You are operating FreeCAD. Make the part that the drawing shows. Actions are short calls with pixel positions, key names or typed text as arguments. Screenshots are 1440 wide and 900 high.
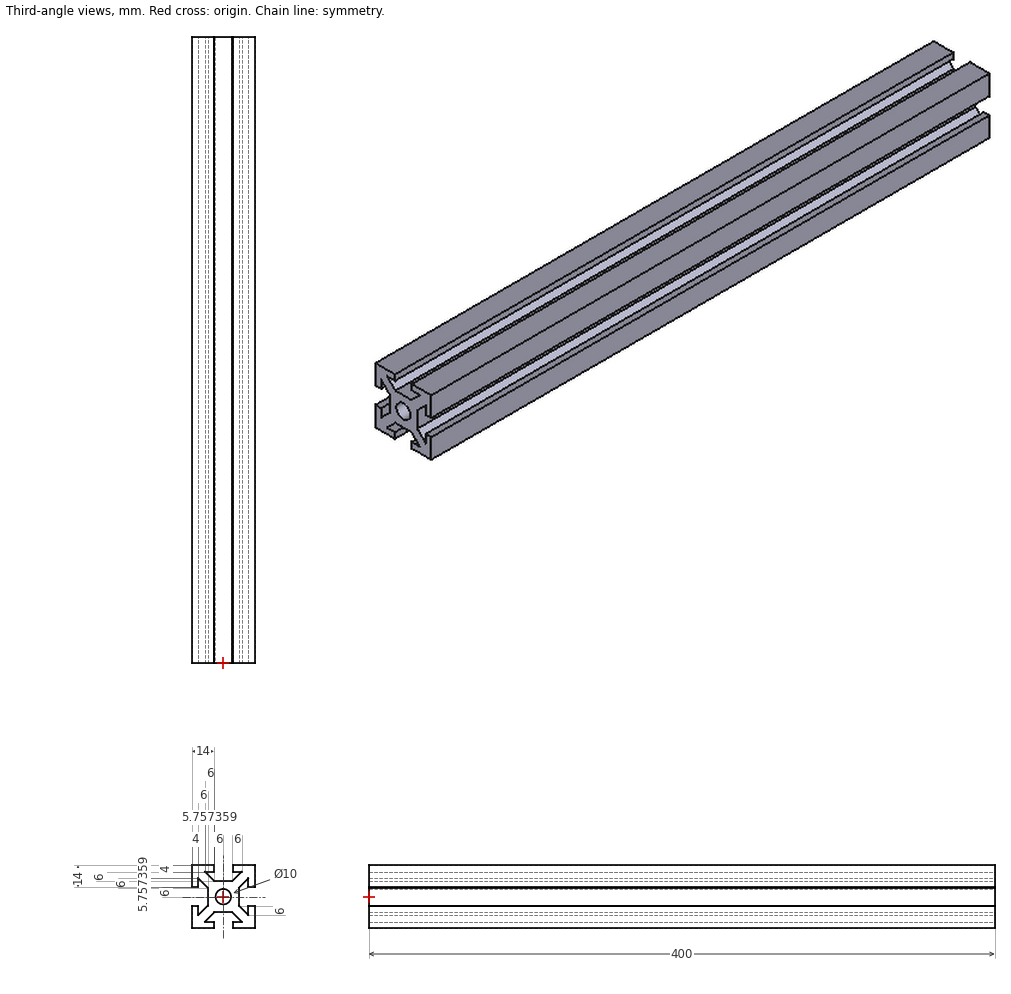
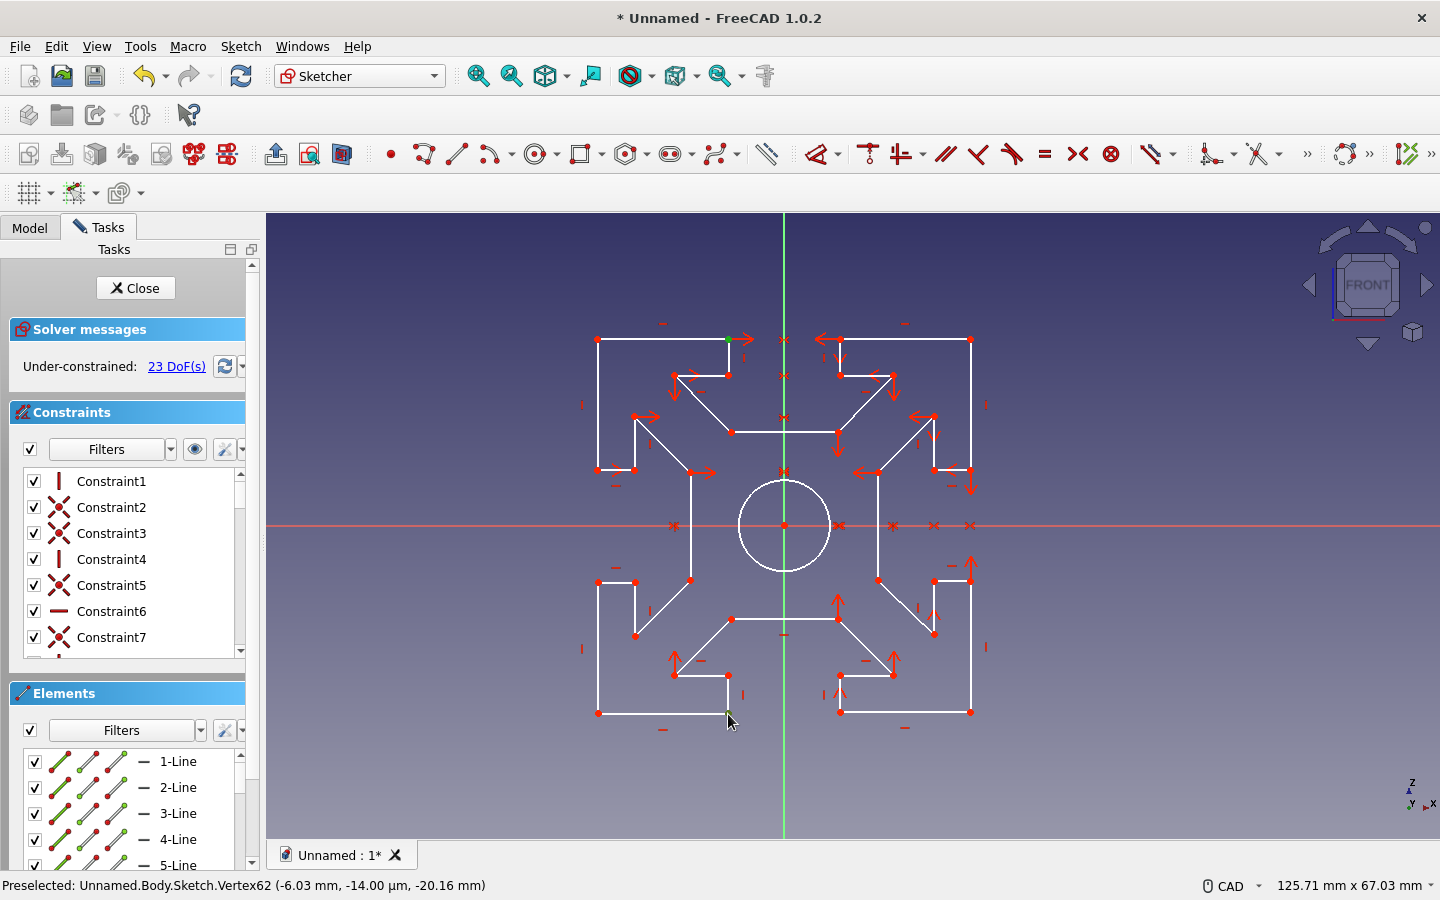
click(364, 526)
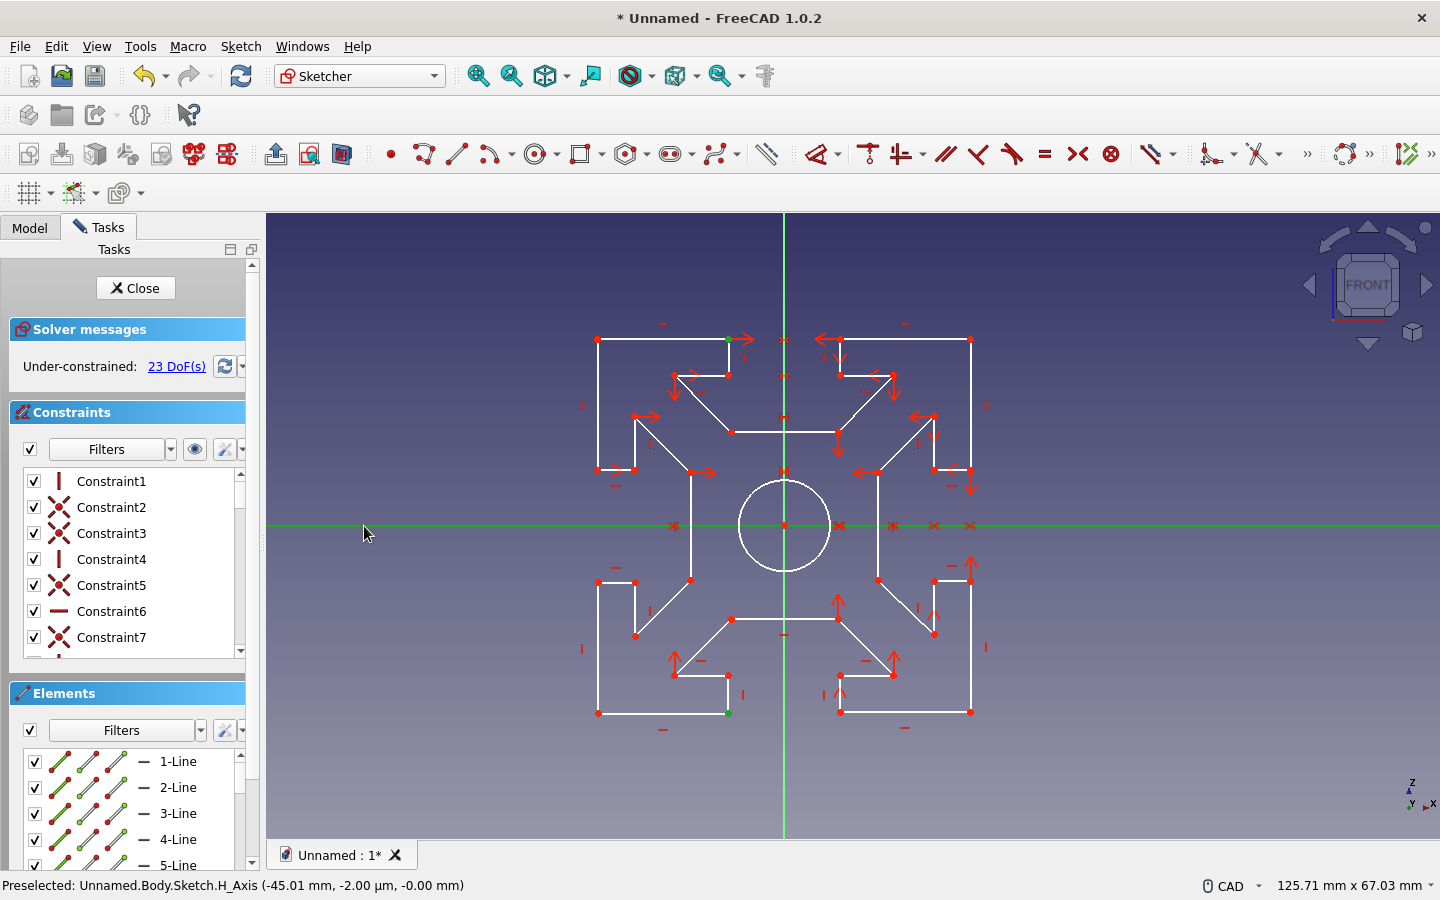
key(s)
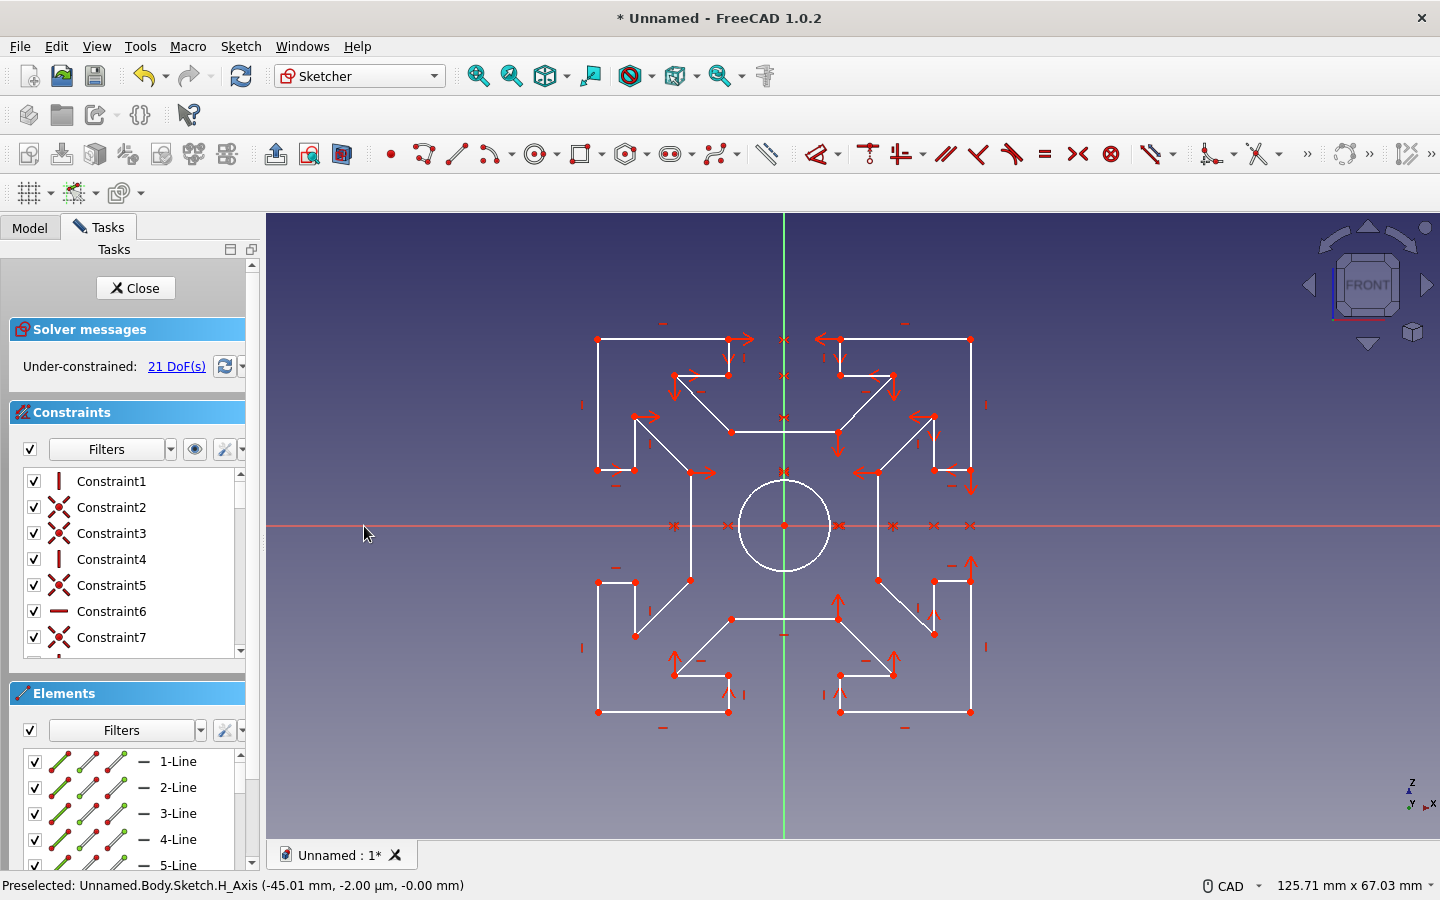
click(598, 470)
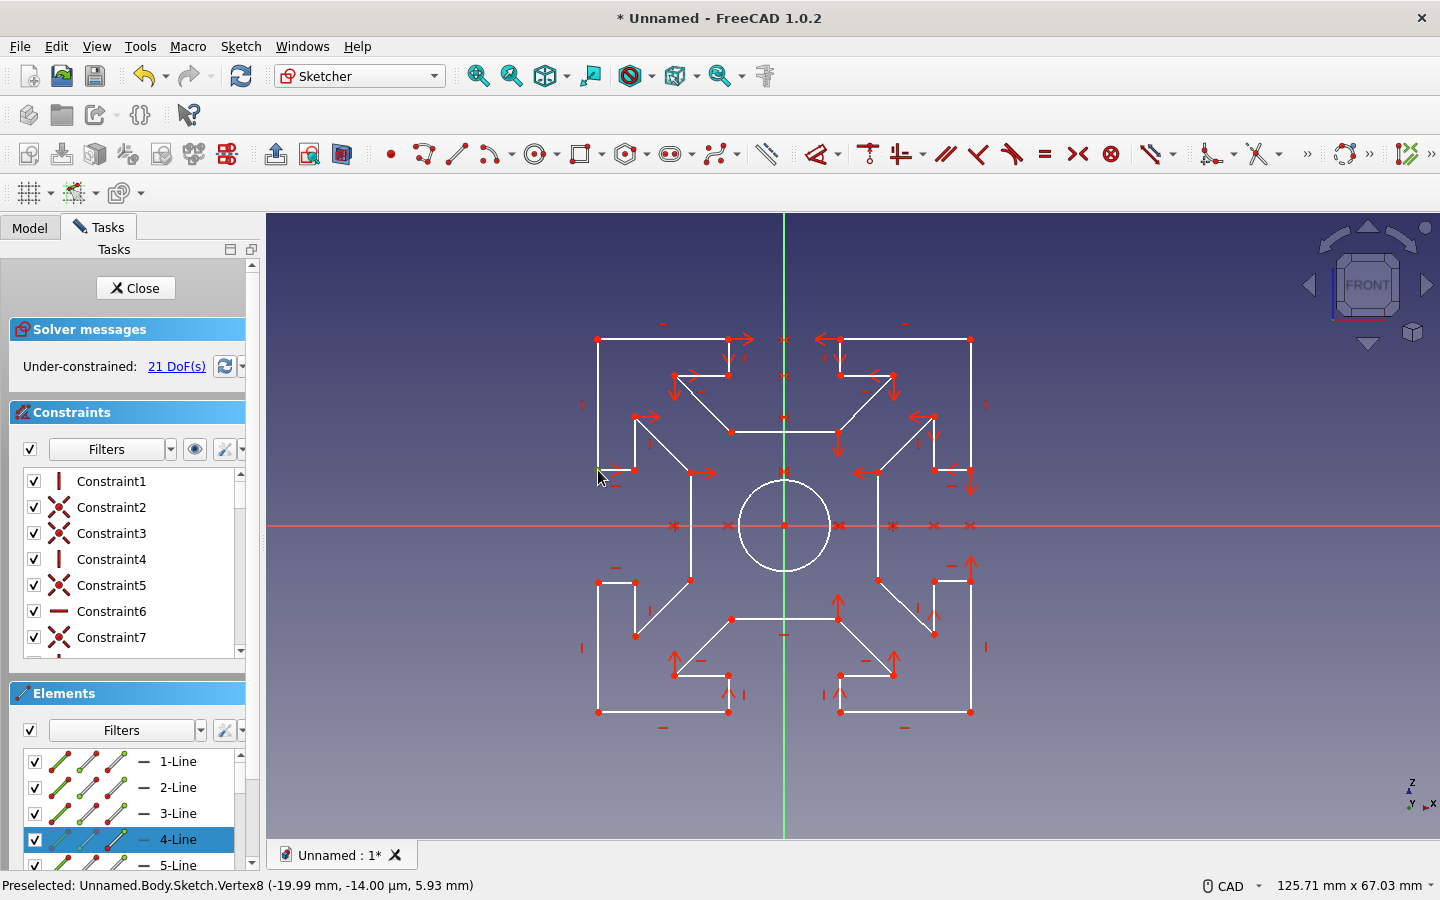
click(598, 583)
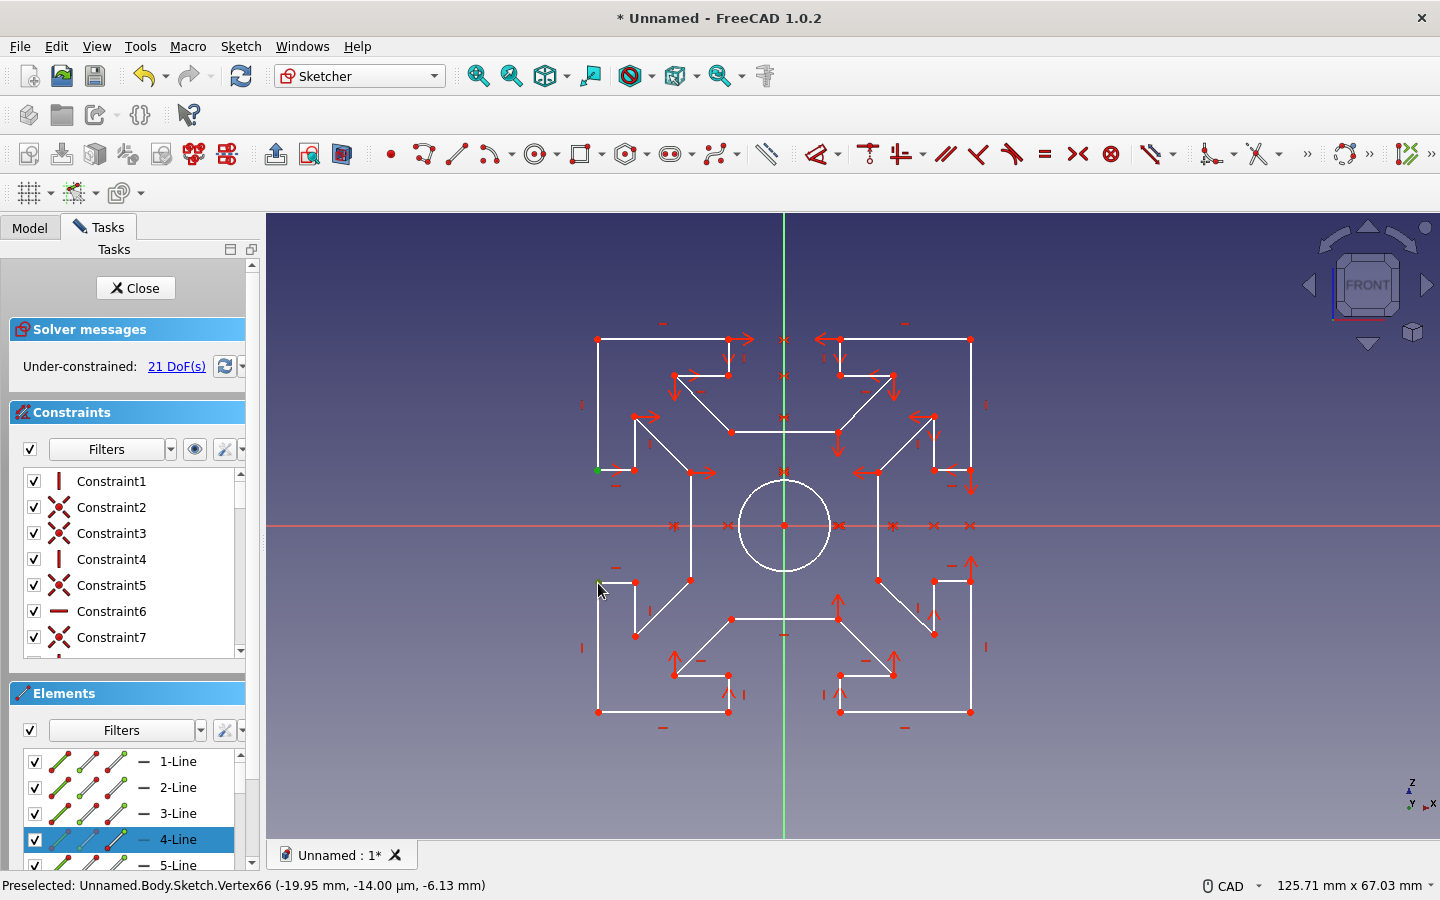
click(364, 526)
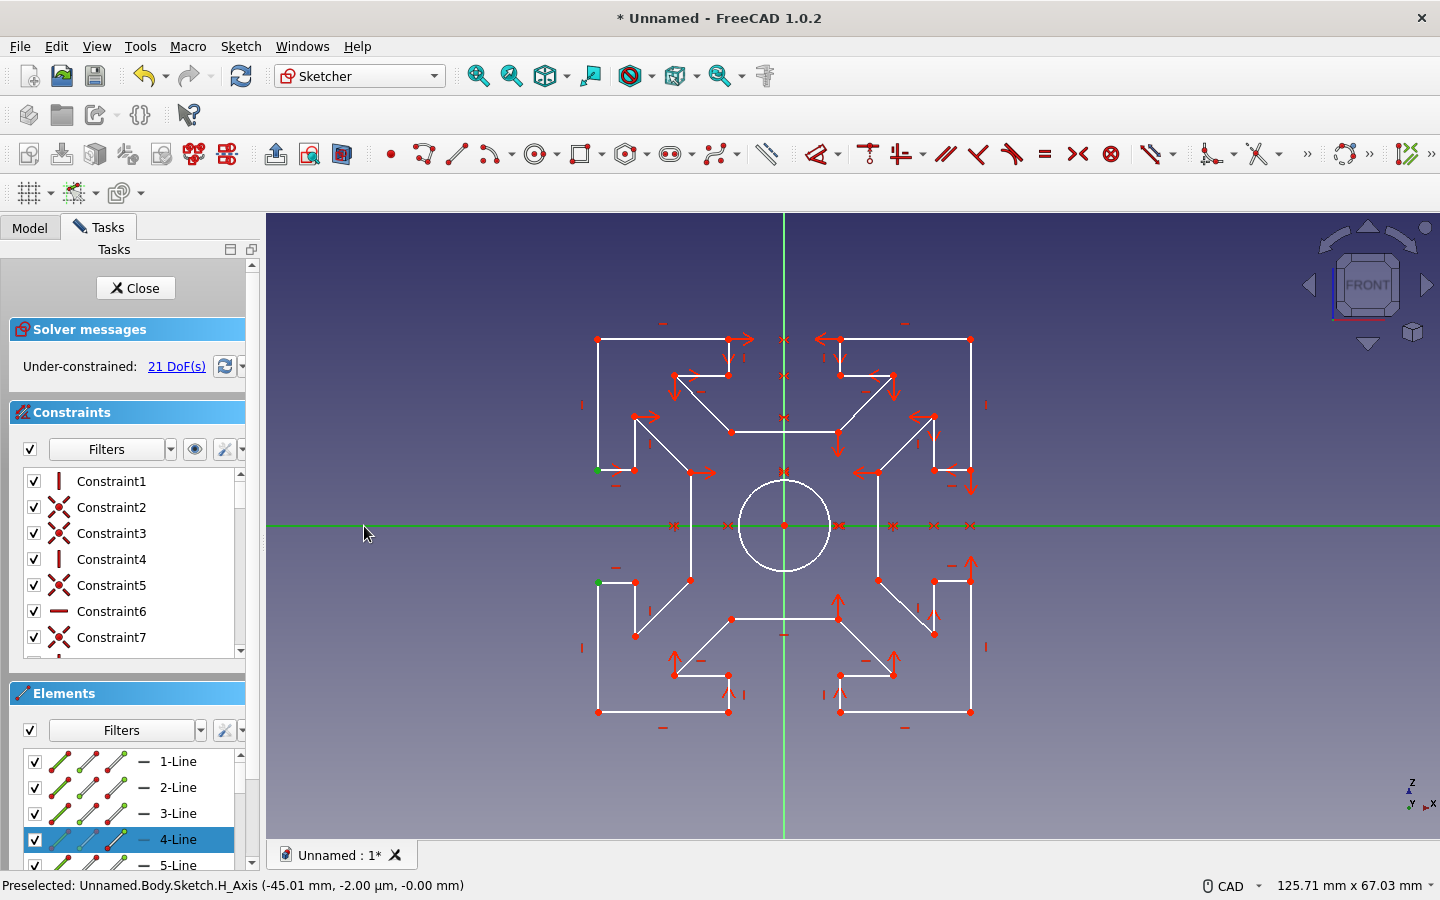
key(s)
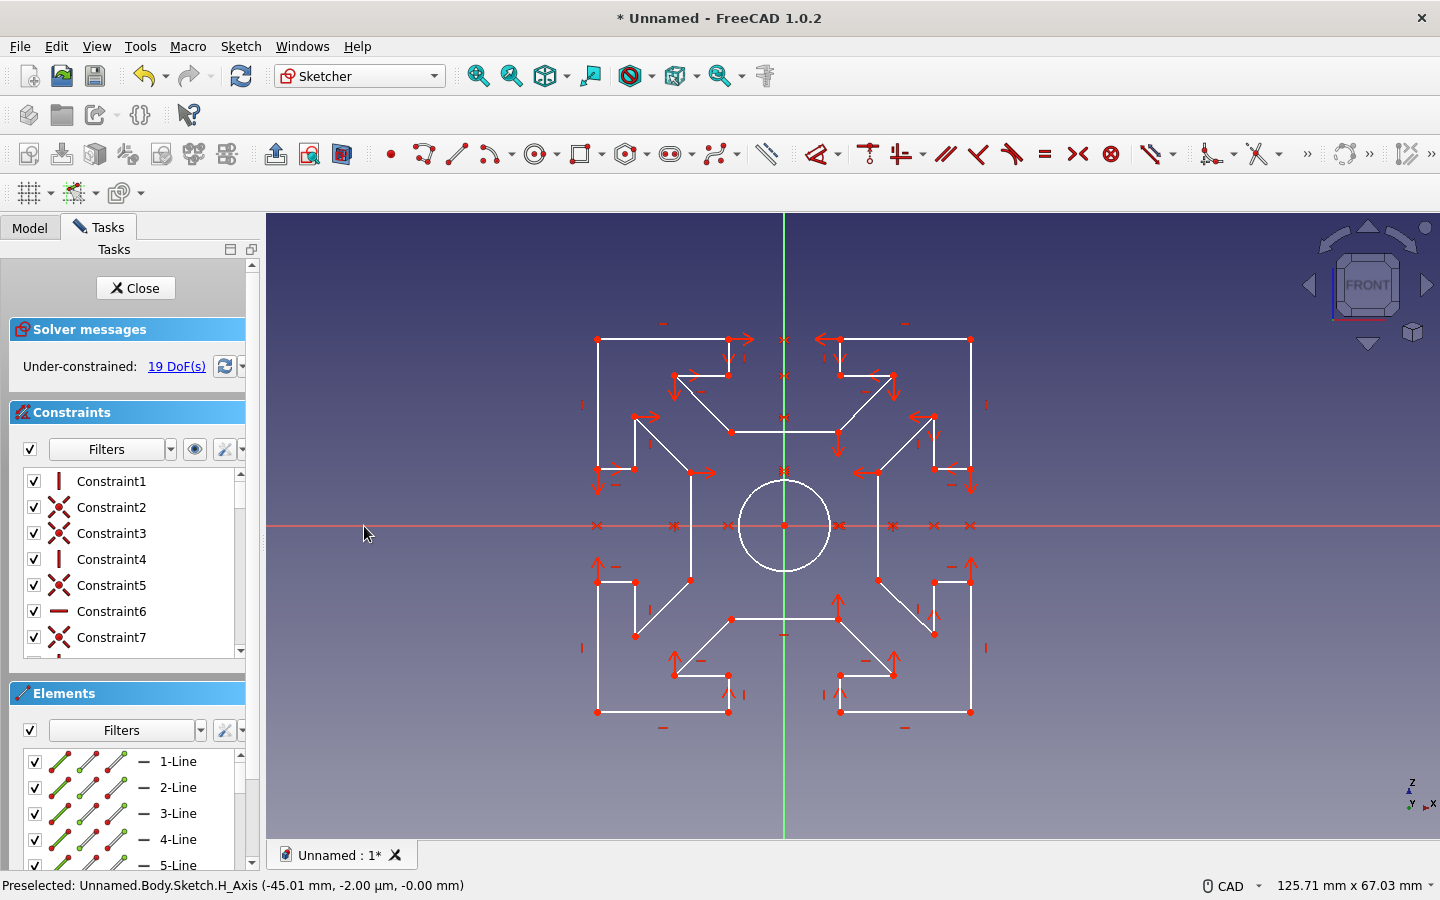
click(635, 417)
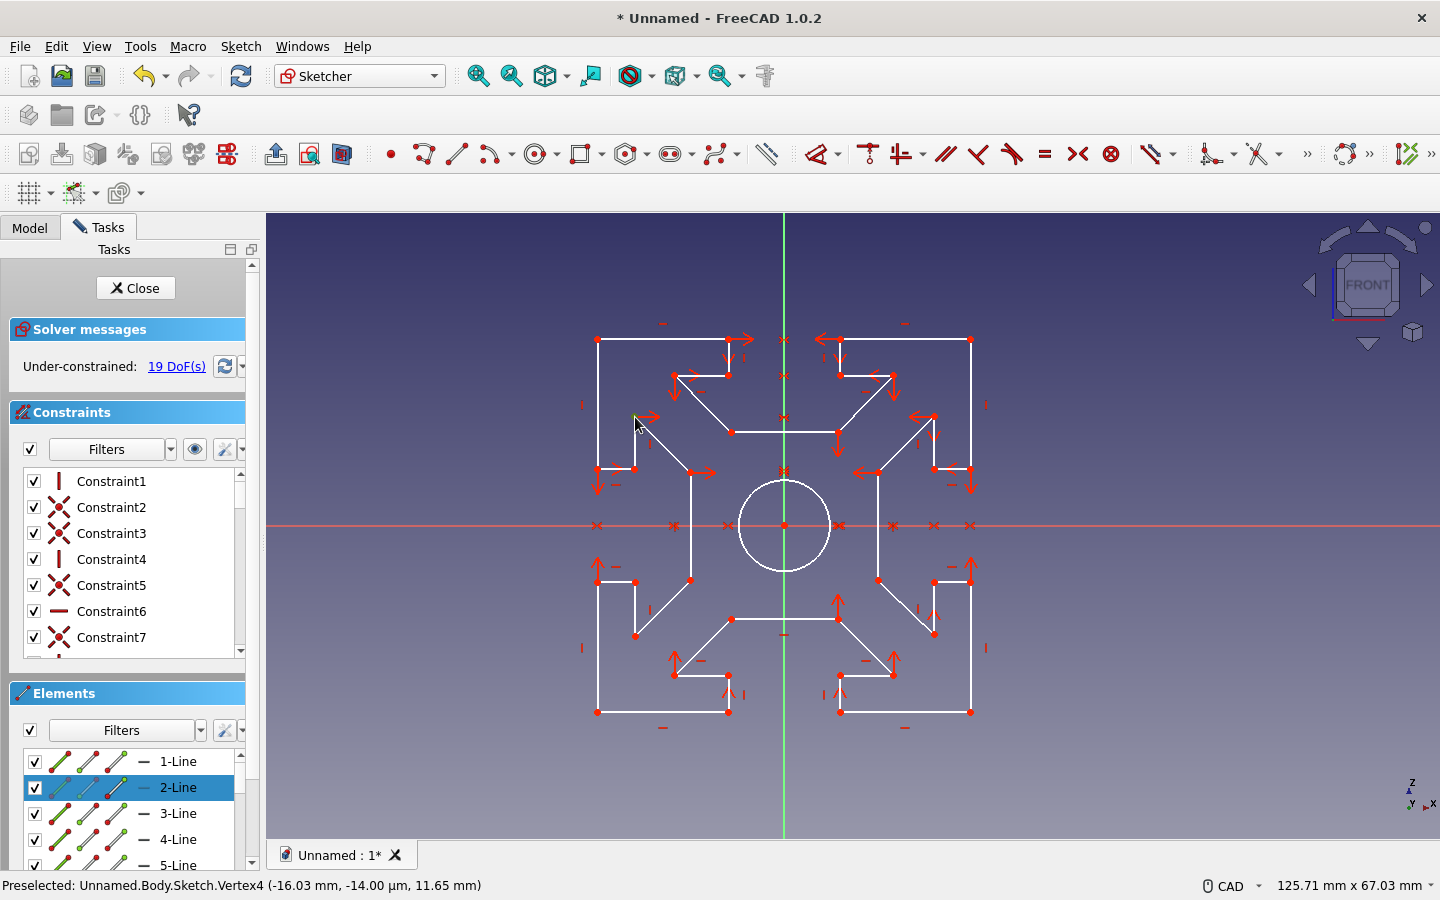
click(635, 637)